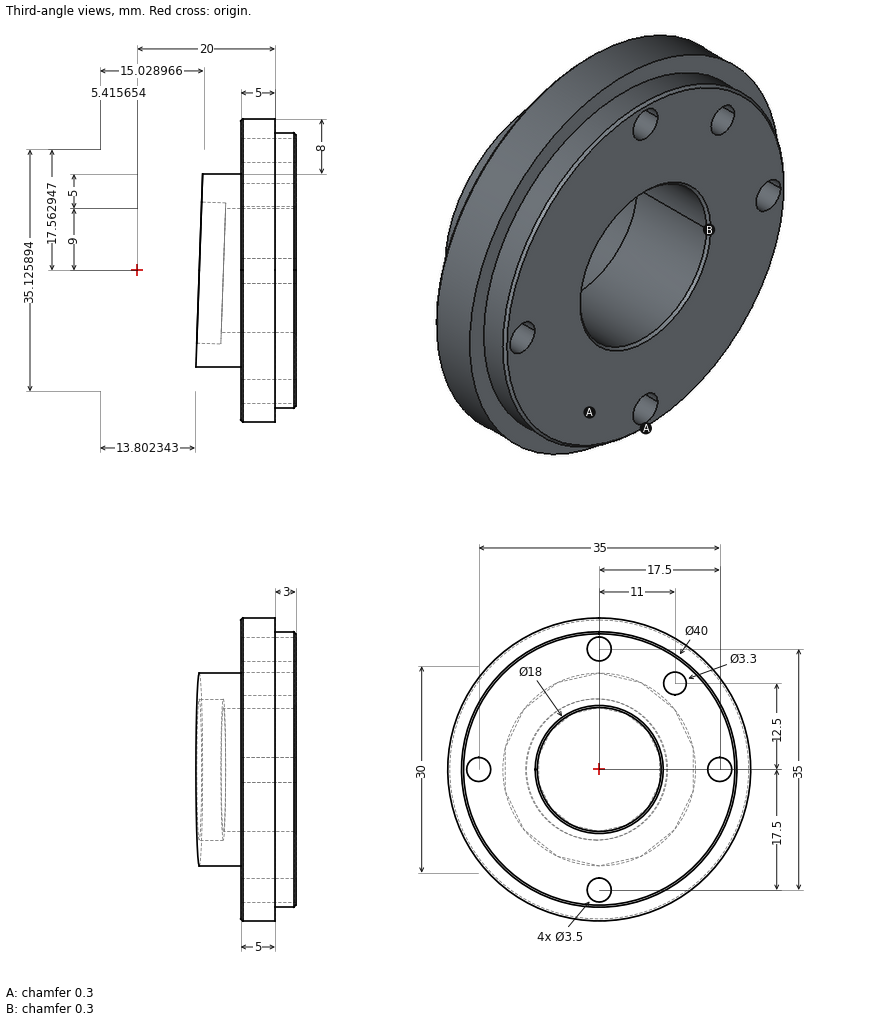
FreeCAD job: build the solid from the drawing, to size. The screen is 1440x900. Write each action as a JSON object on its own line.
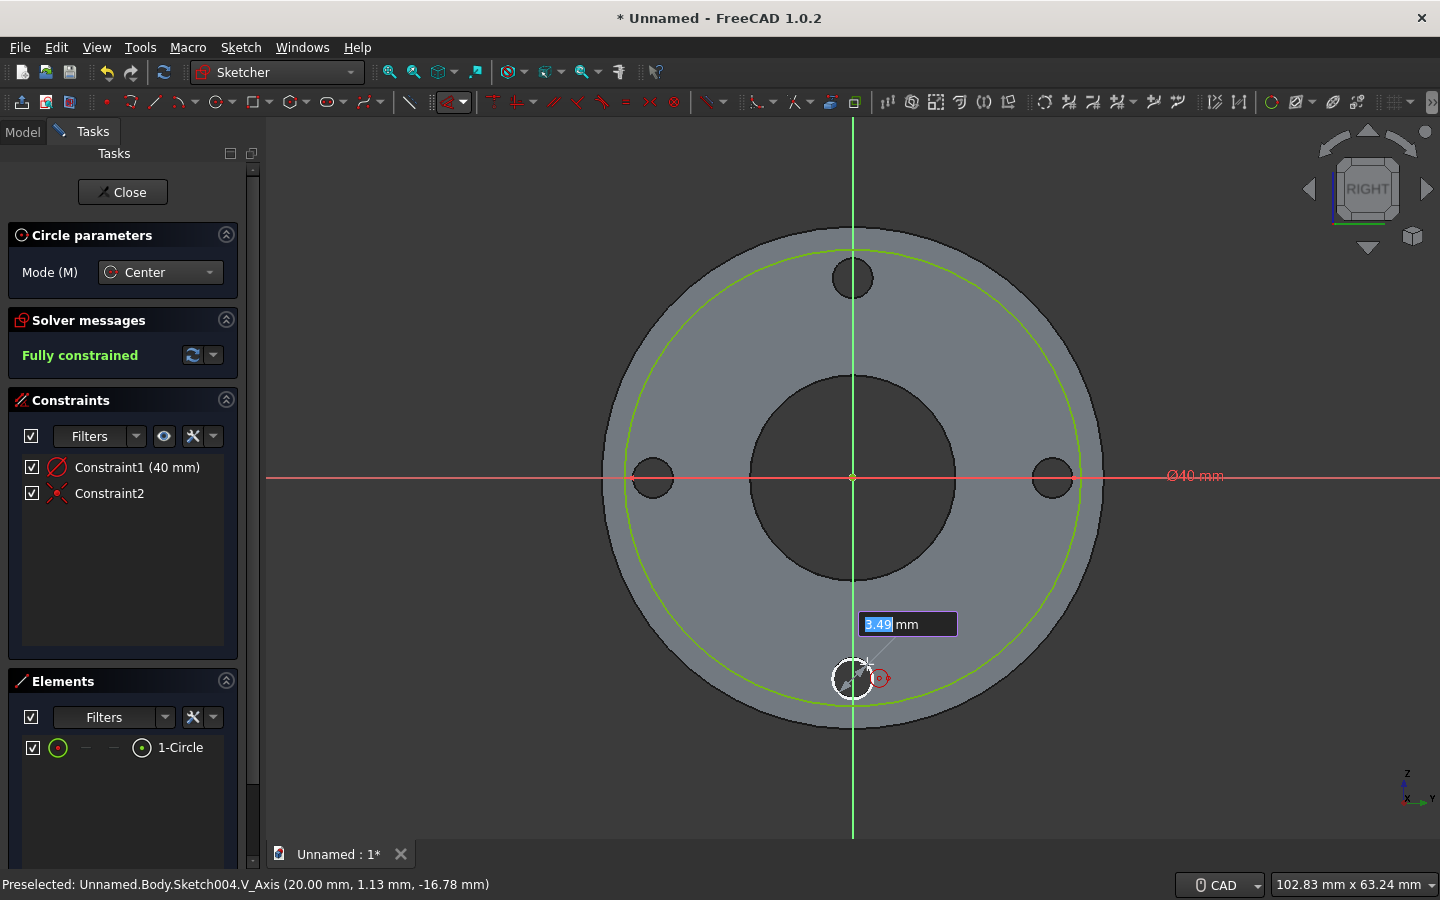
{"action": "type", "text": "3.5"}
{"action": "key", "text": "Return"}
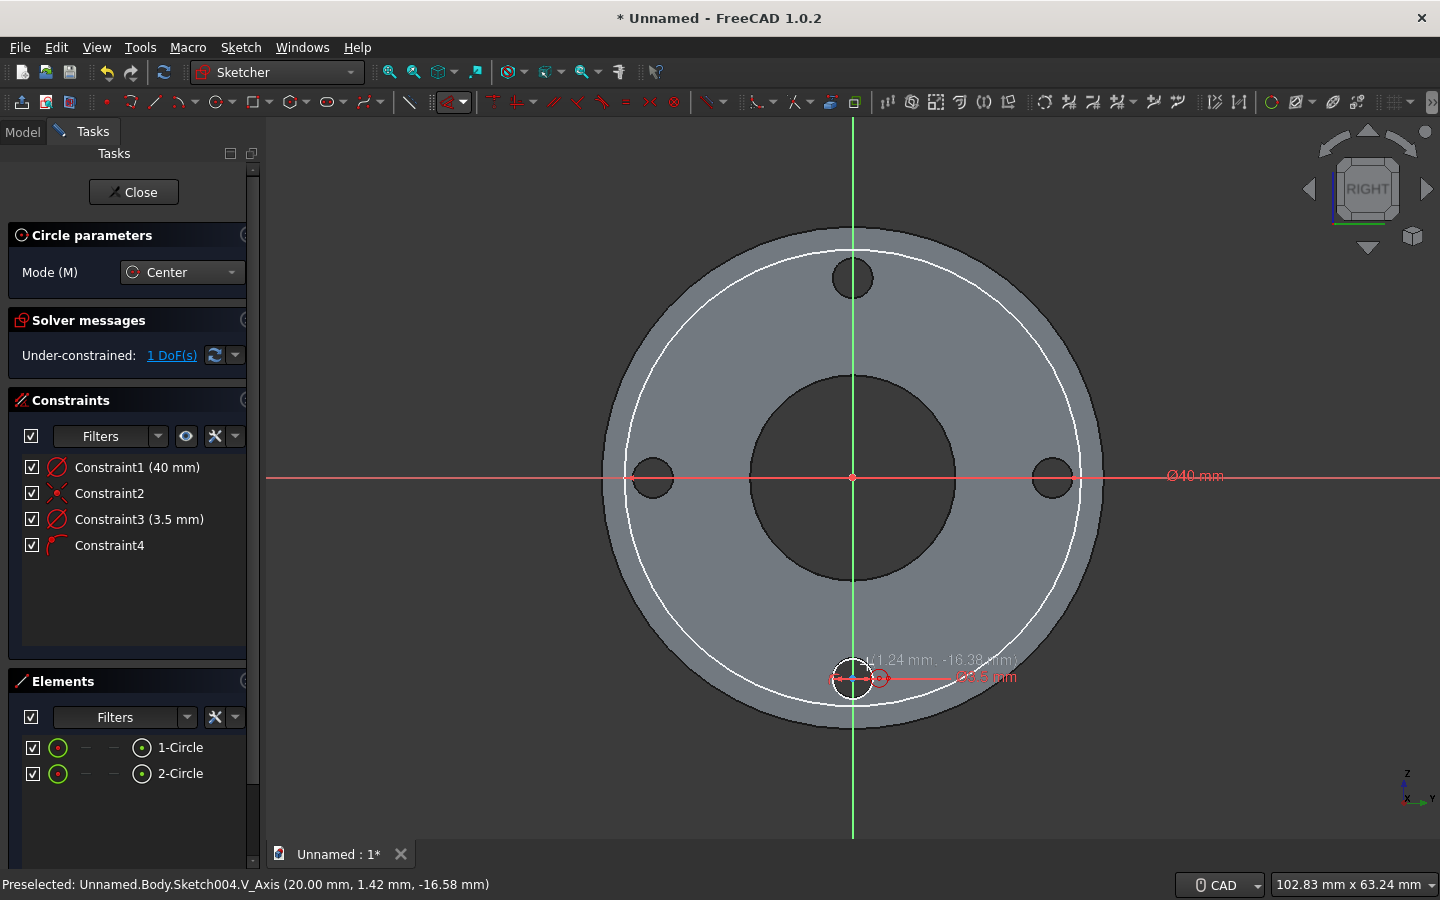
{"action": "left_click", "coordinate": [1053, 478]}
{"action": "mouse_move", "coordinate": [1038, 464]}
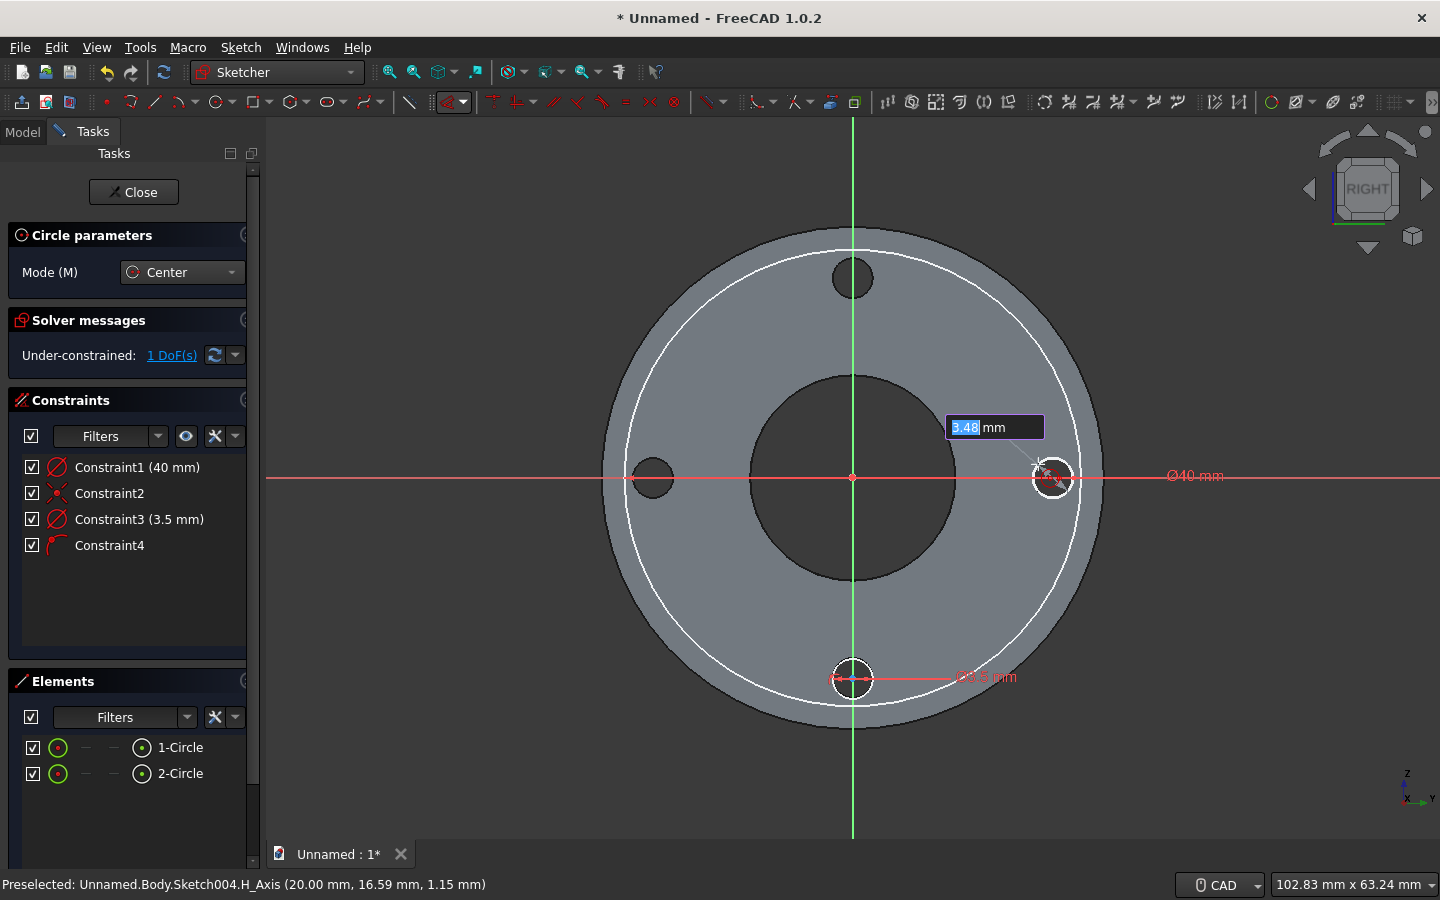
{"action": "type", "text": "3.5"}
{"action": "key", "text": "Return"}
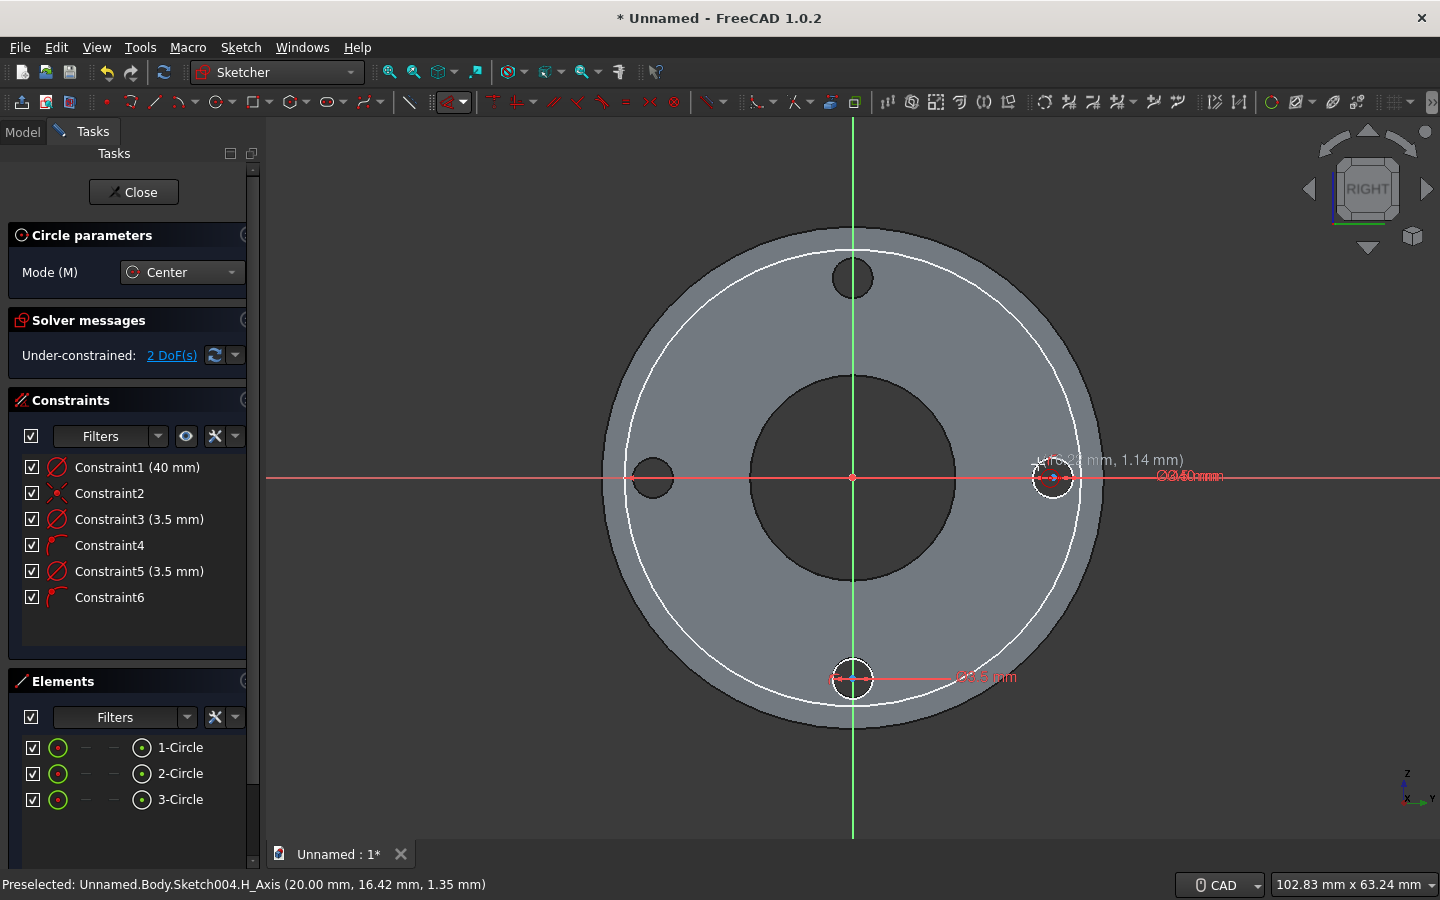
{"action": "left_click", "coordinate": [853, 478]}
{"action": "mouse_move", "coordinate": [925, 405]}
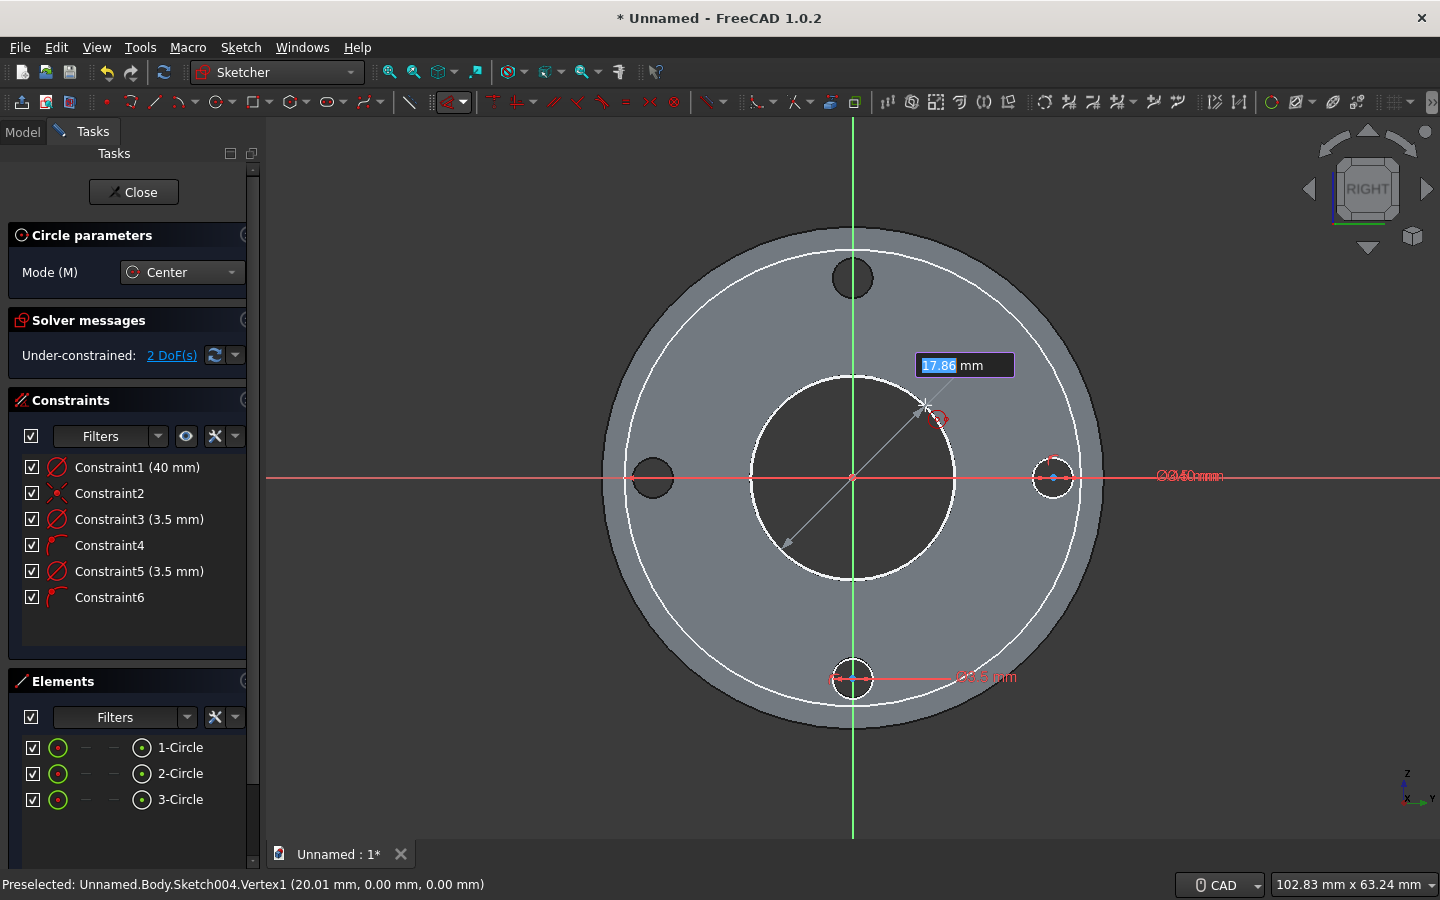
{"action": "type", "text": "18"}
{"action": "key", "text": "Return"}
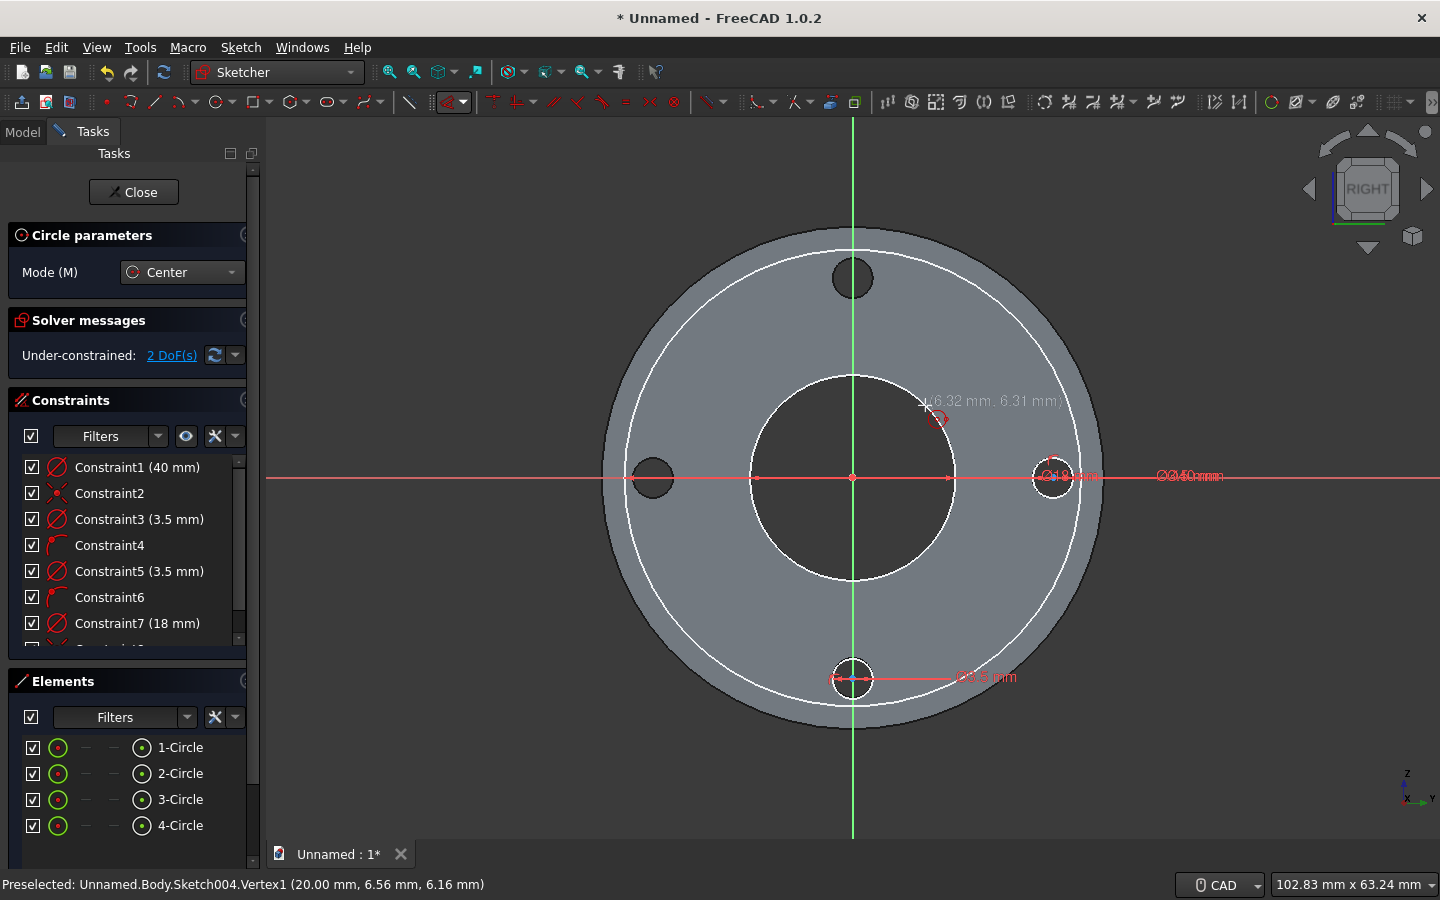
{"action": "left_click", "coordinate": [853, 278]}
{"action": "mouse_move", "coordinate": [867, 292]}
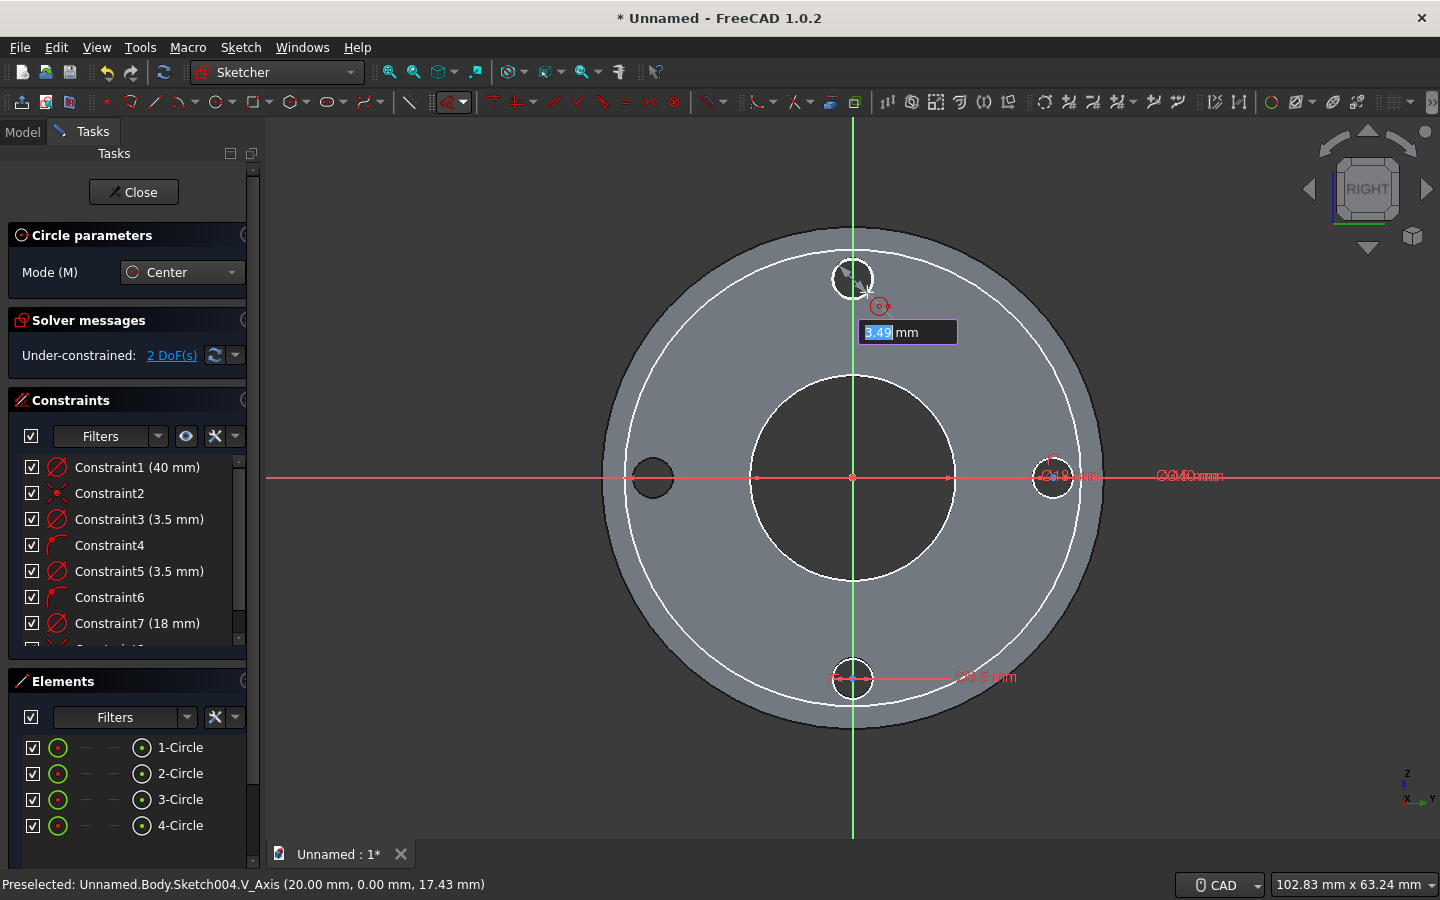
{"action": "type", "text": "3.5"}
{"action": "key", "text": "Return"}